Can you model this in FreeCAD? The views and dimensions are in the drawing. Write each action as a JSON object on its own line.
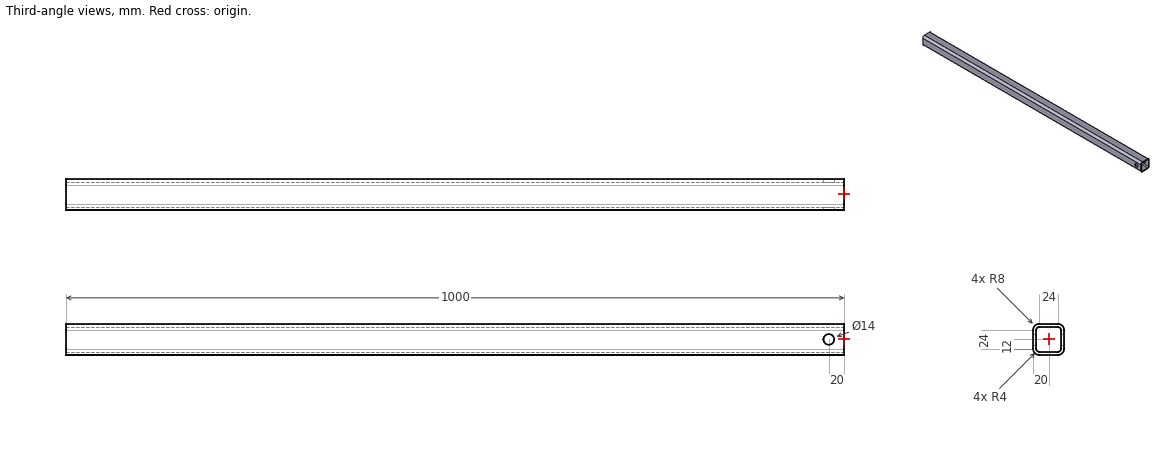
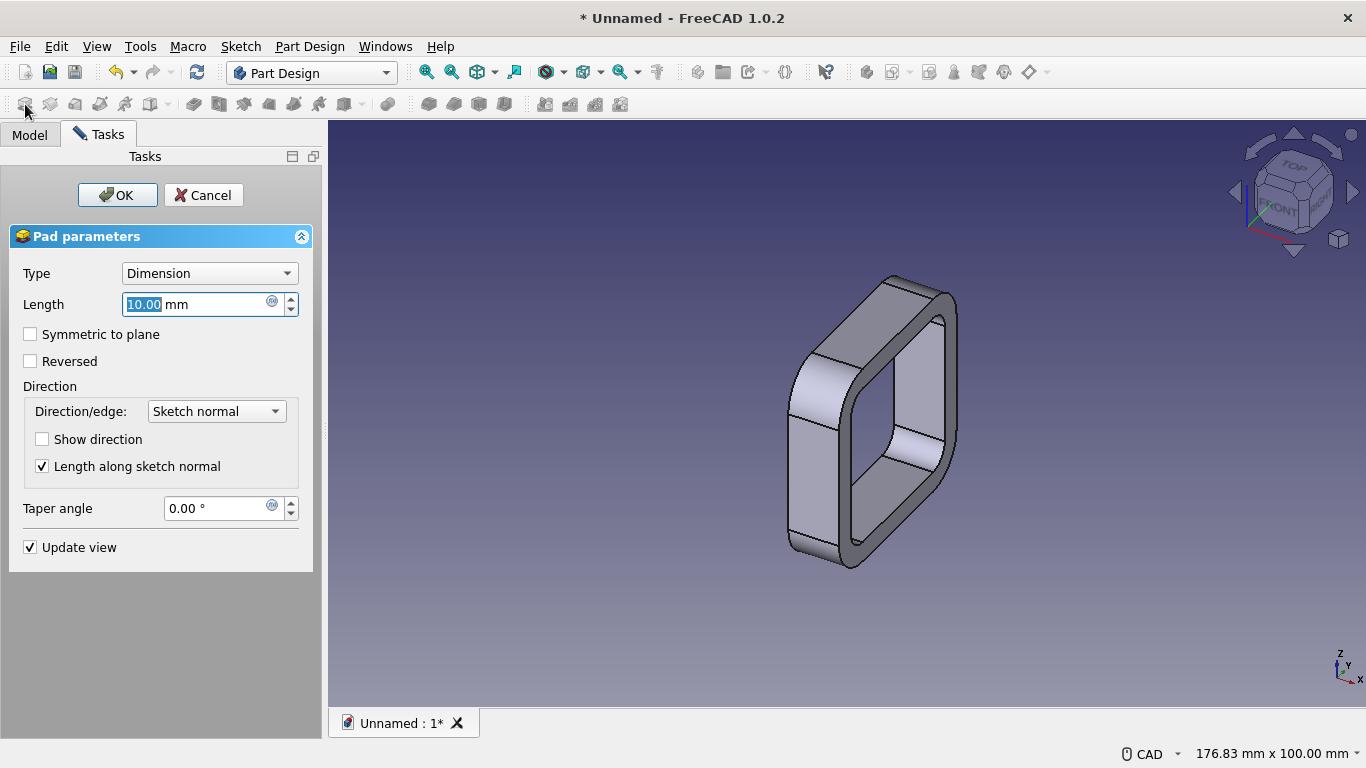
{"action": "type", "text": "1000"}
{"action": "key", "text": "Tab"}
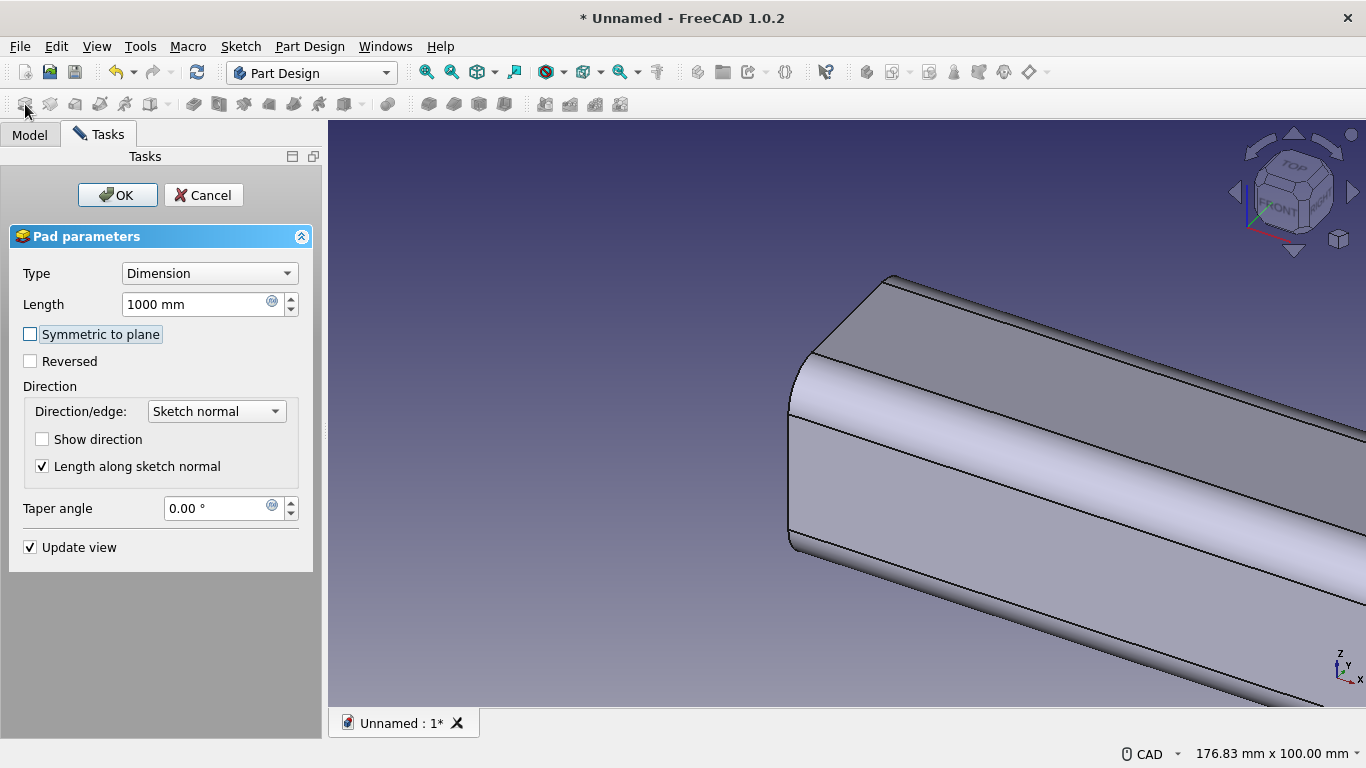
{"action": "left_click", "coordinate": [31, 361]}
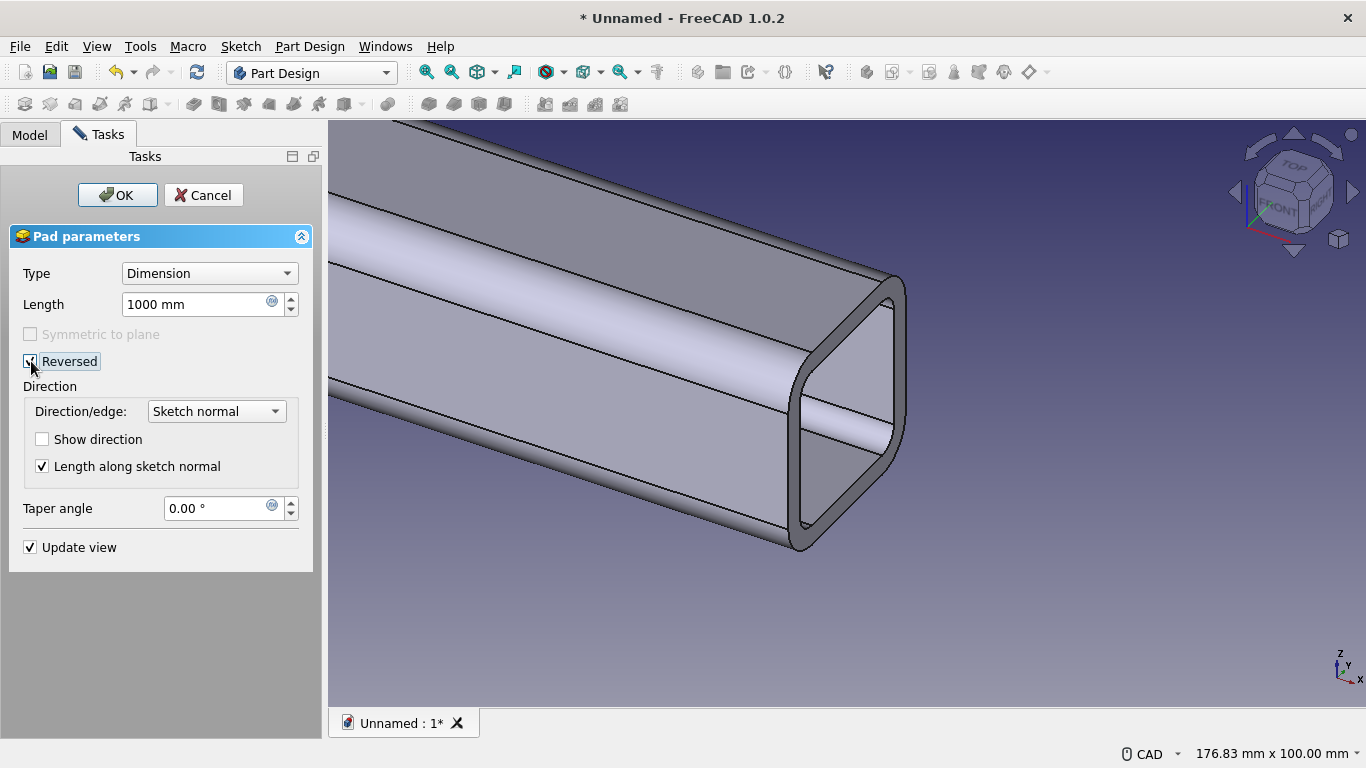
{"action": "left_click", "coordinate": [118, 195]}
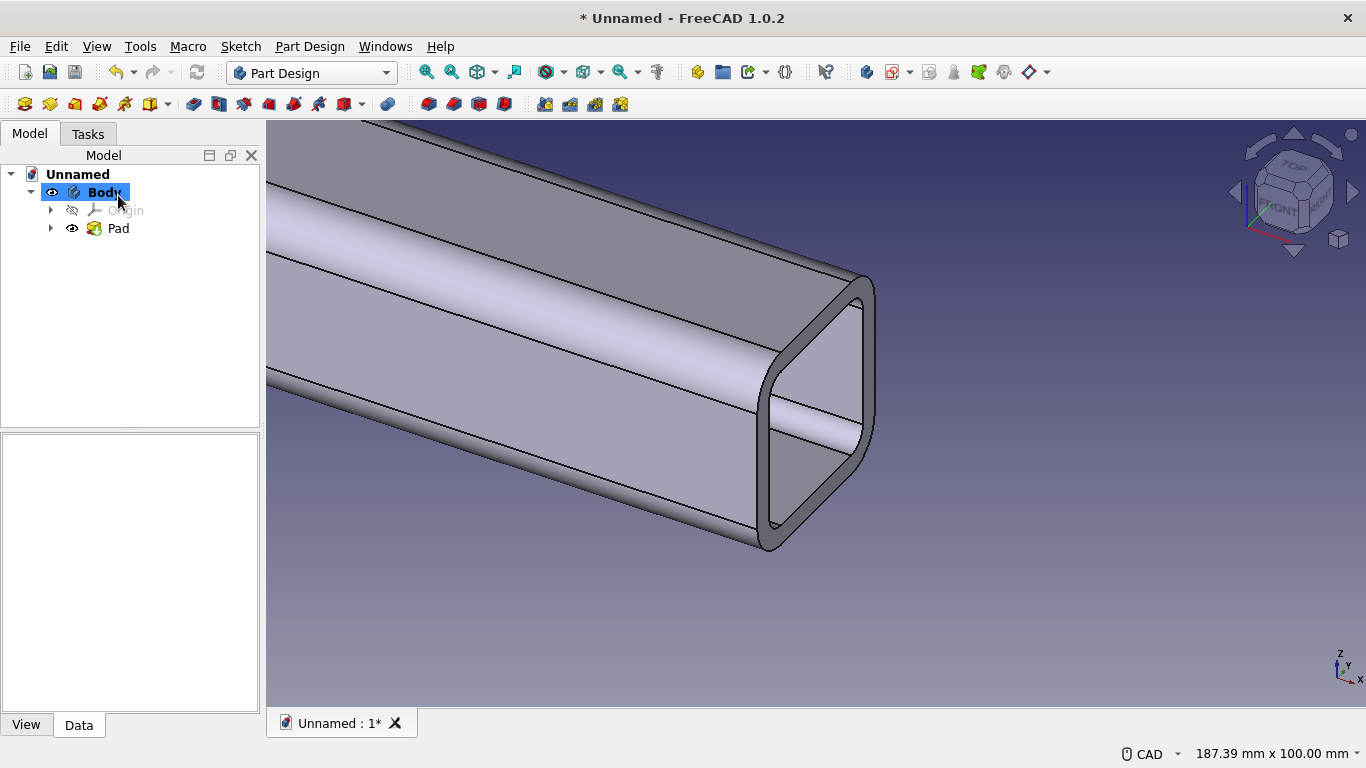
{"action": "left_click", "coordinate": [427, 72]}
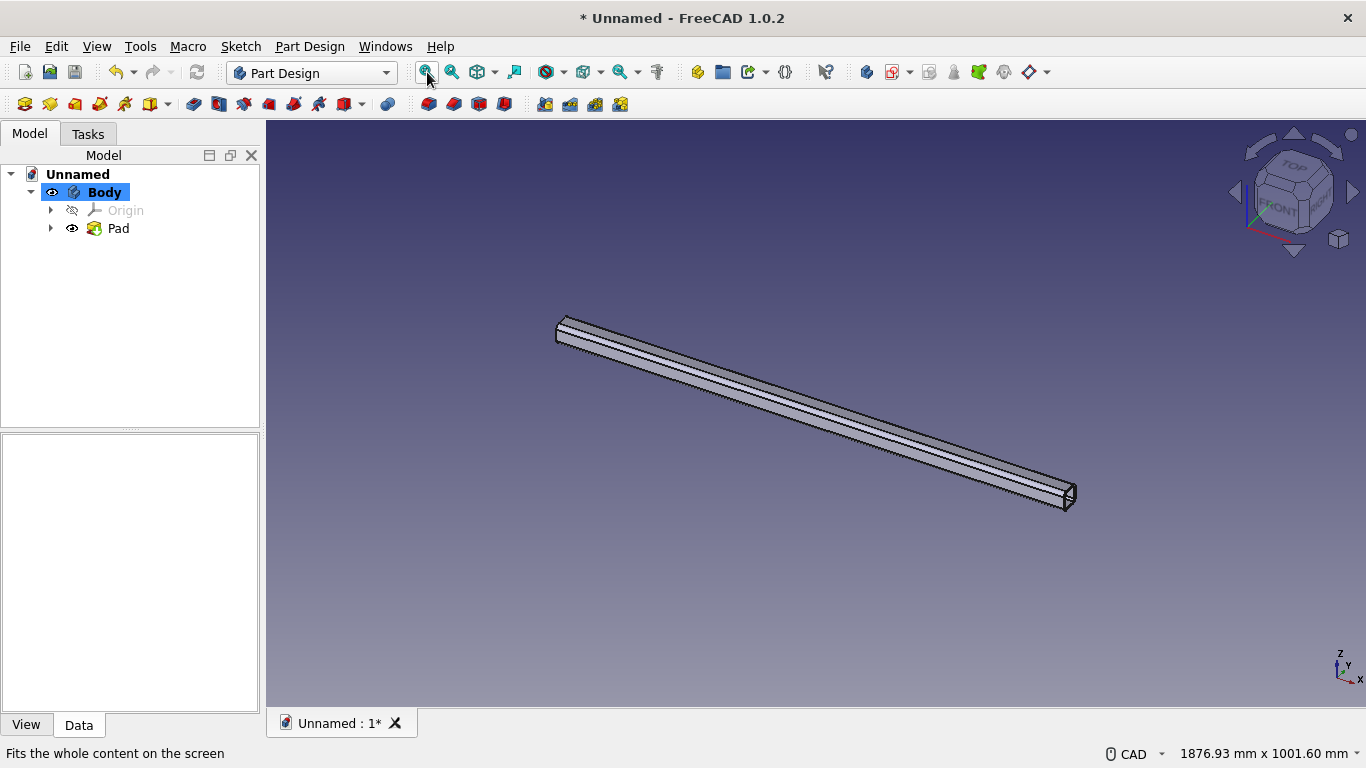
{"action": "key", "text": "4"}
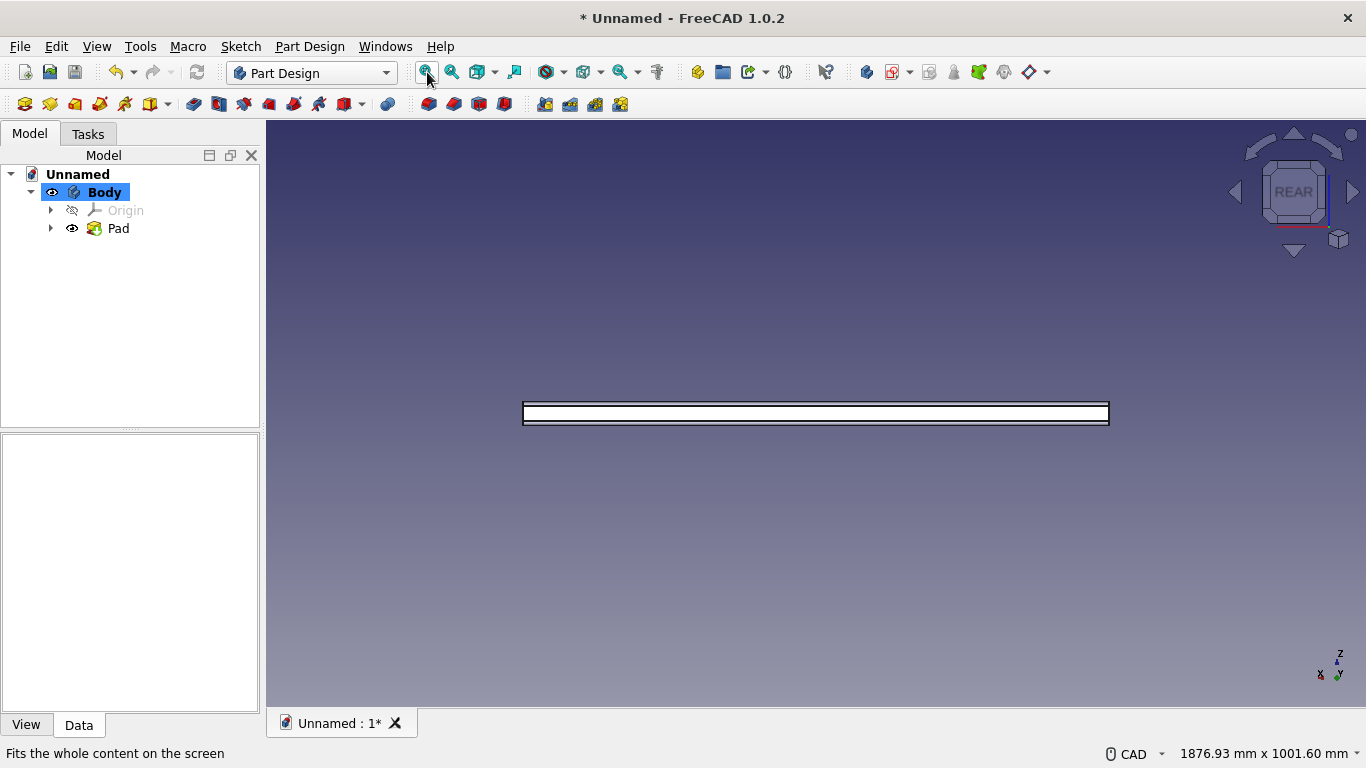
{"action": "key", "text": "3"}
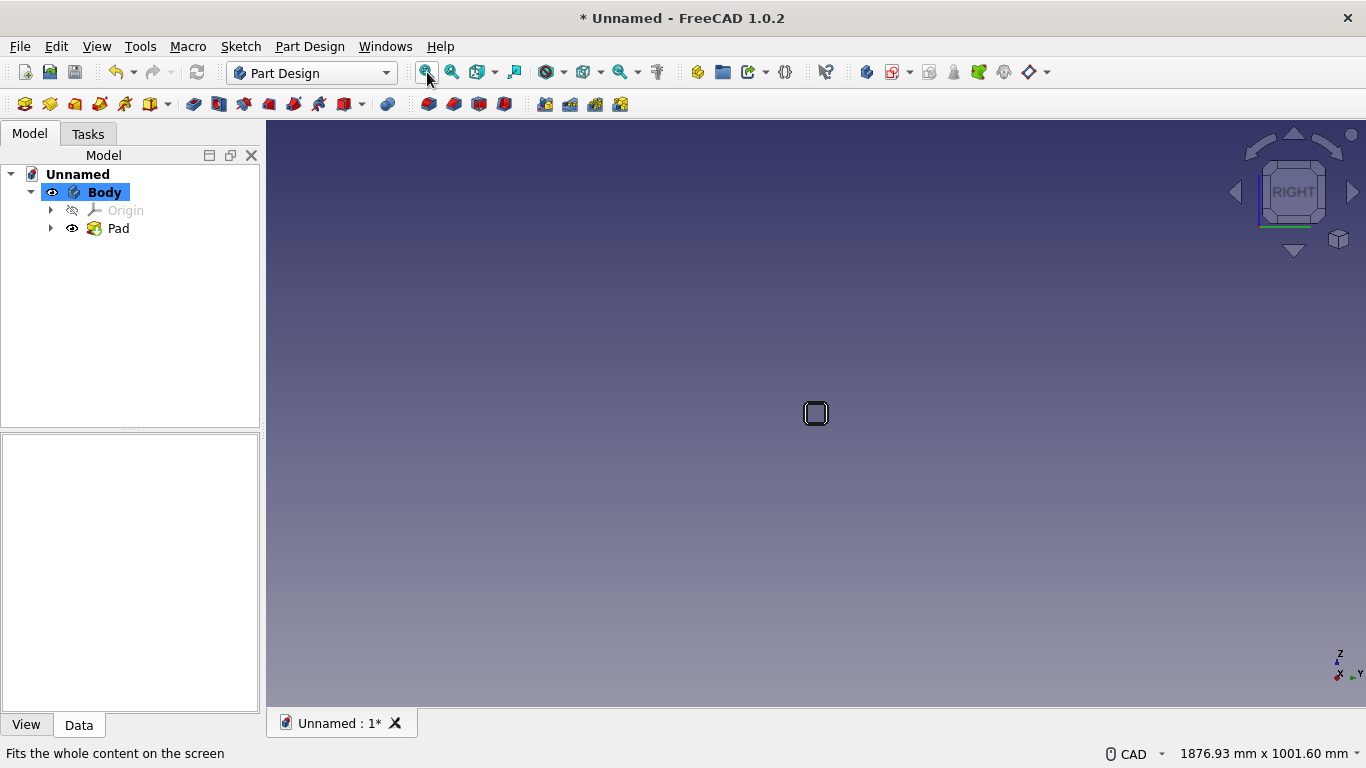
{"action": "left_click", "coordinate": [427, 72]}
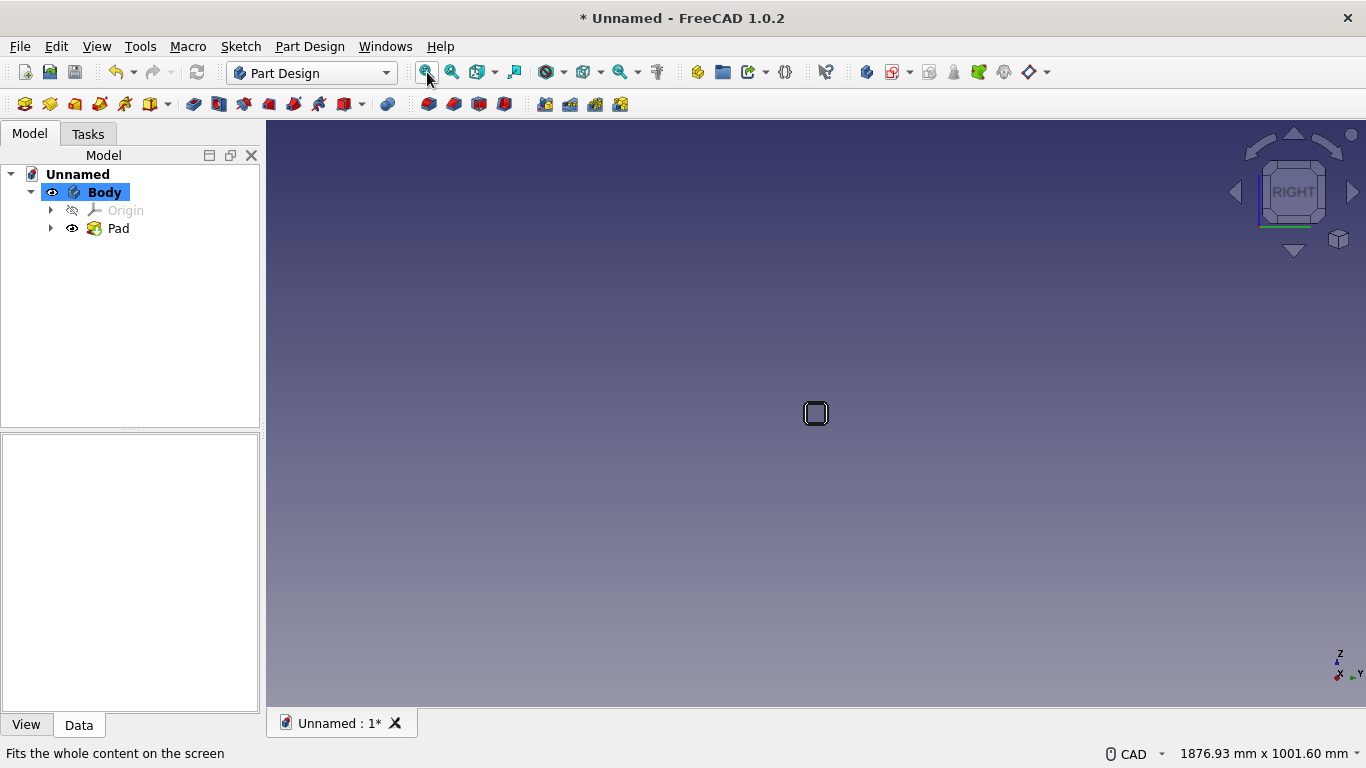
{"action": "key", "text": "5"}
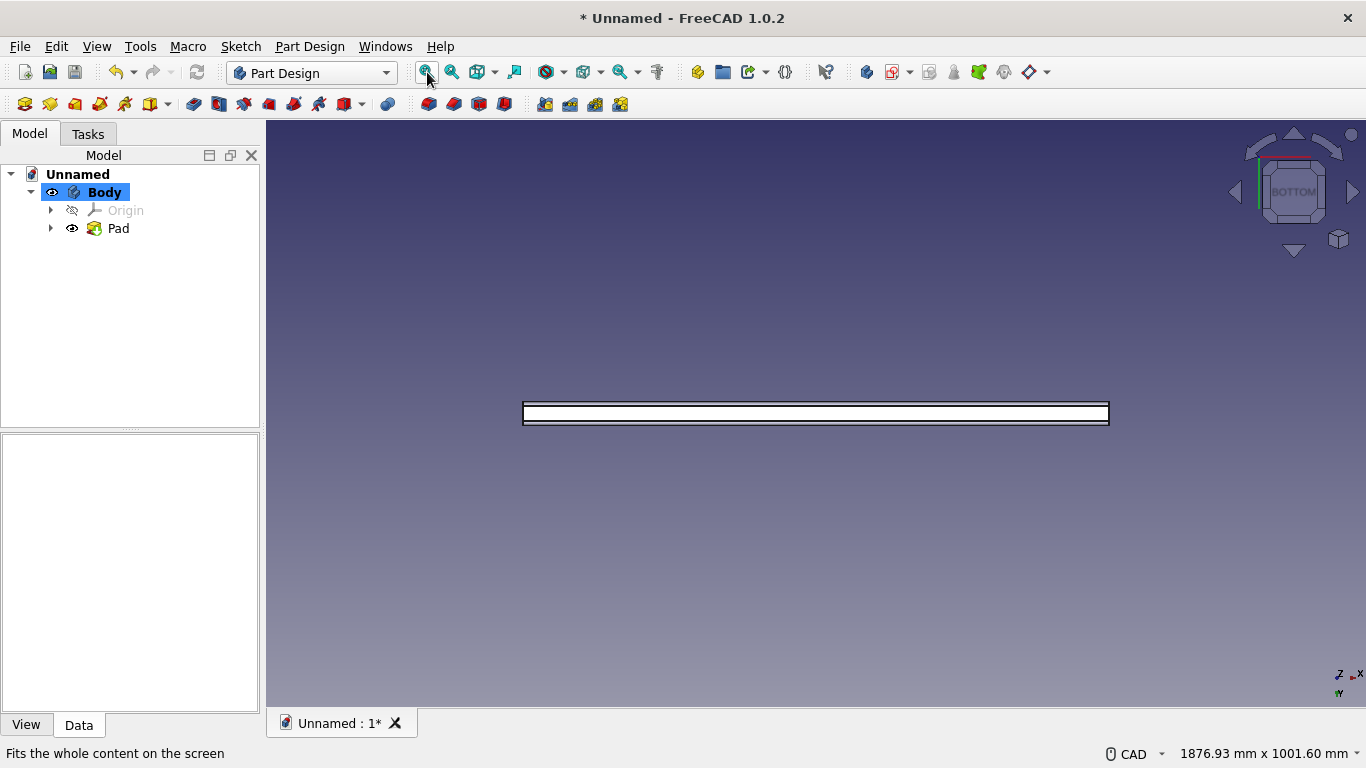
{"action": "left_click", "coordinate": [51, 210]}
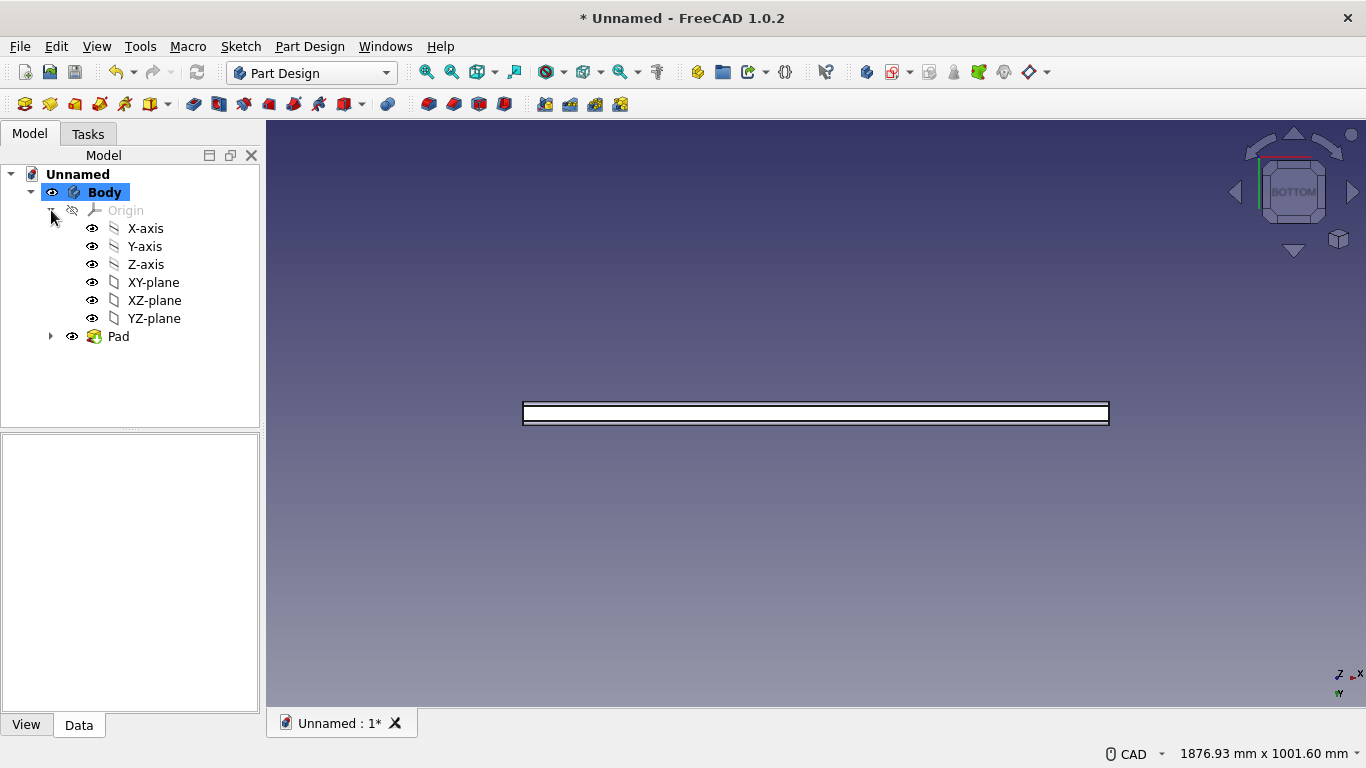
{"action": "left_click", "coordinate": [137, 300]}